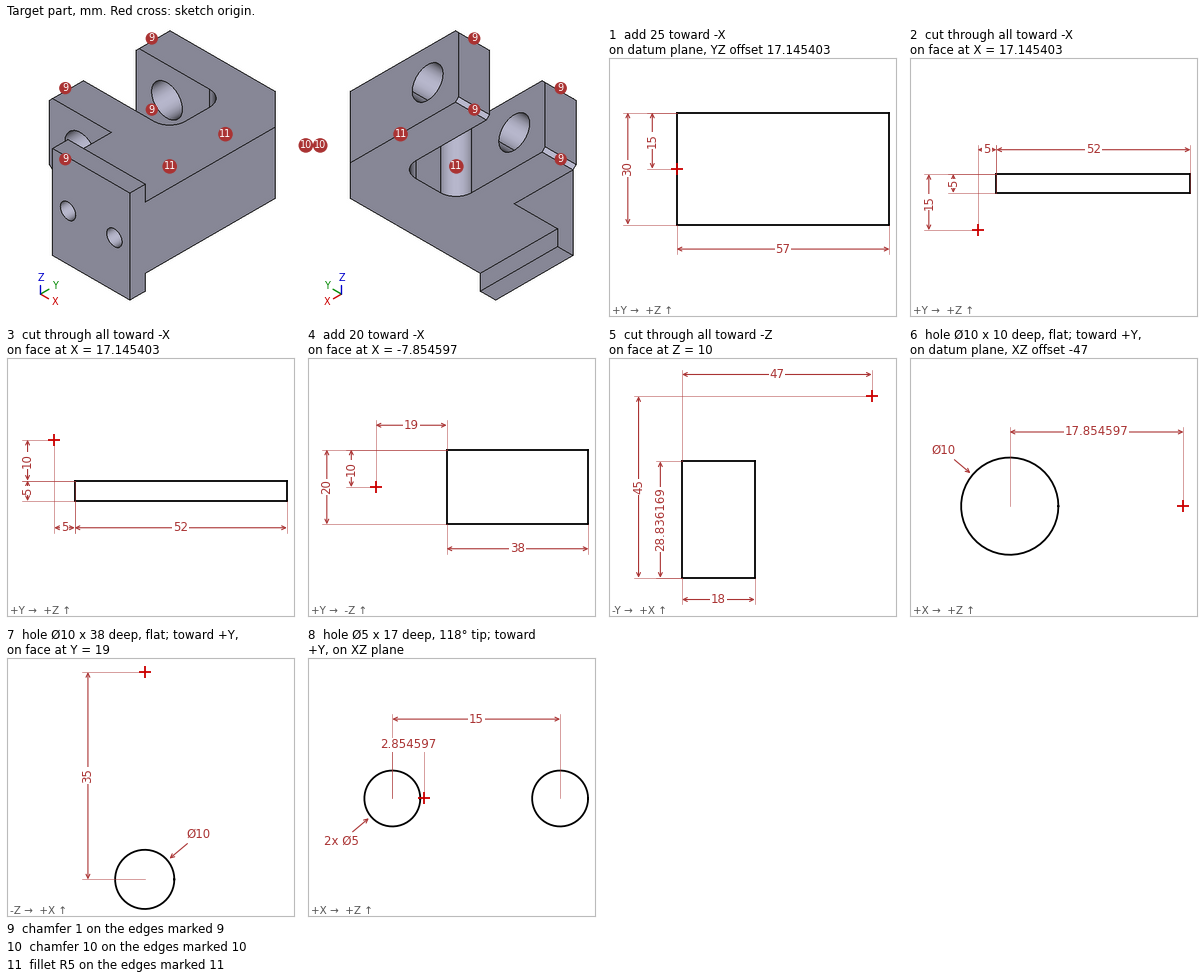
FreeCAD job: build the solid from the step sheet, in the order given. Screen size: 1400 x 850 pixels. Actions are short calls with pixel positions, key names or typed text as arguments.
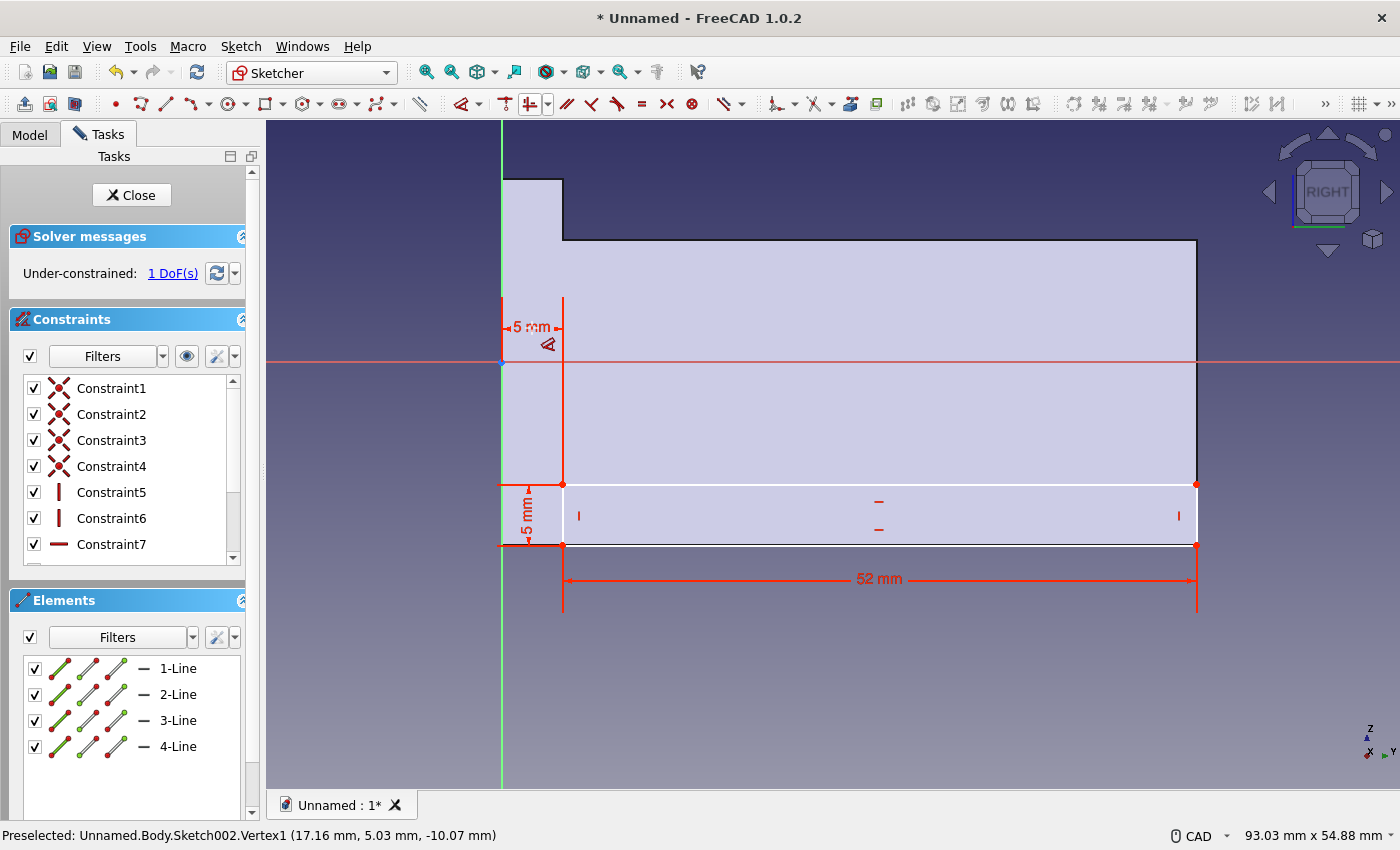
click(563, 485)
click(468, 424)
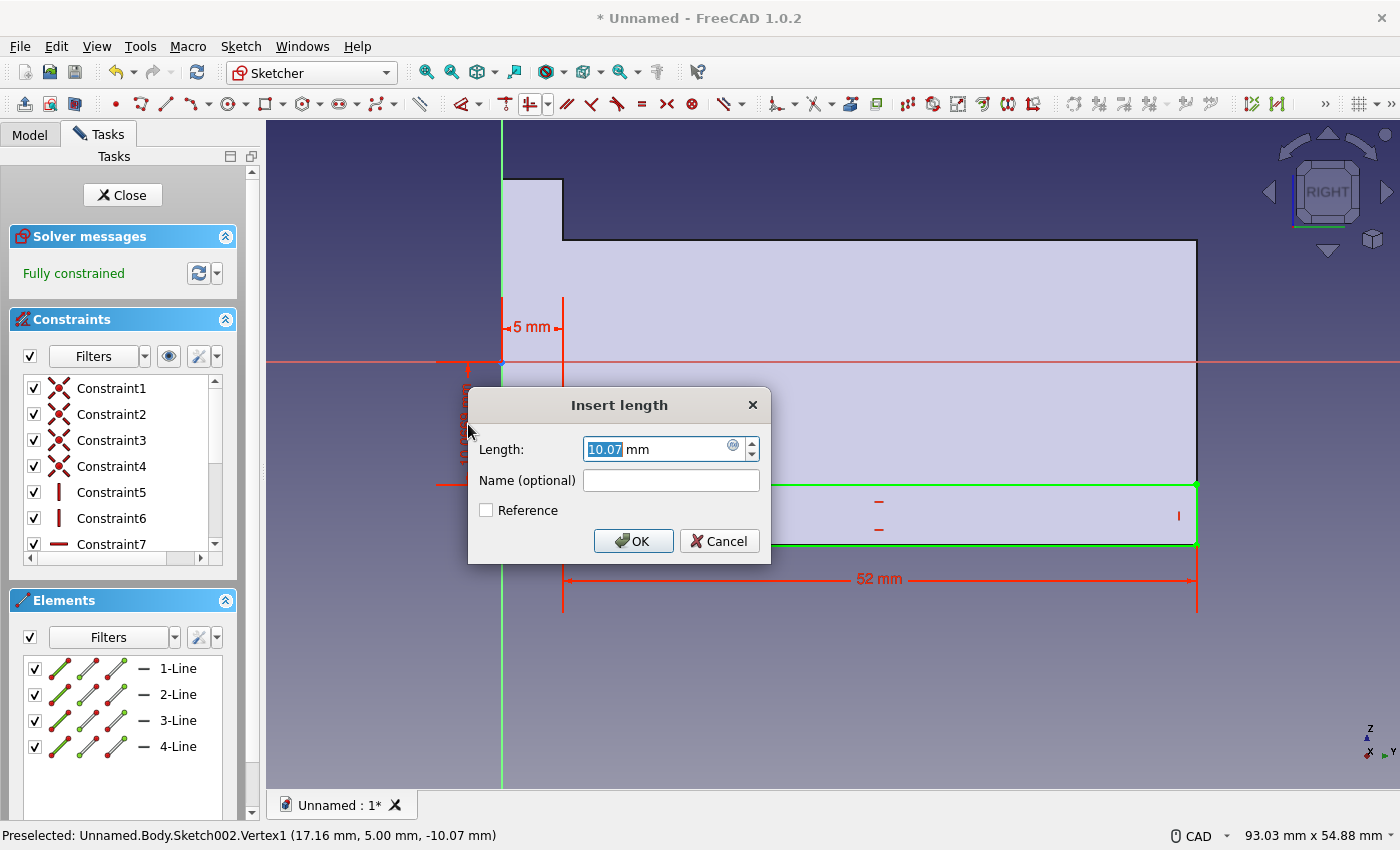
text(10)
key(Return)
key(Escape)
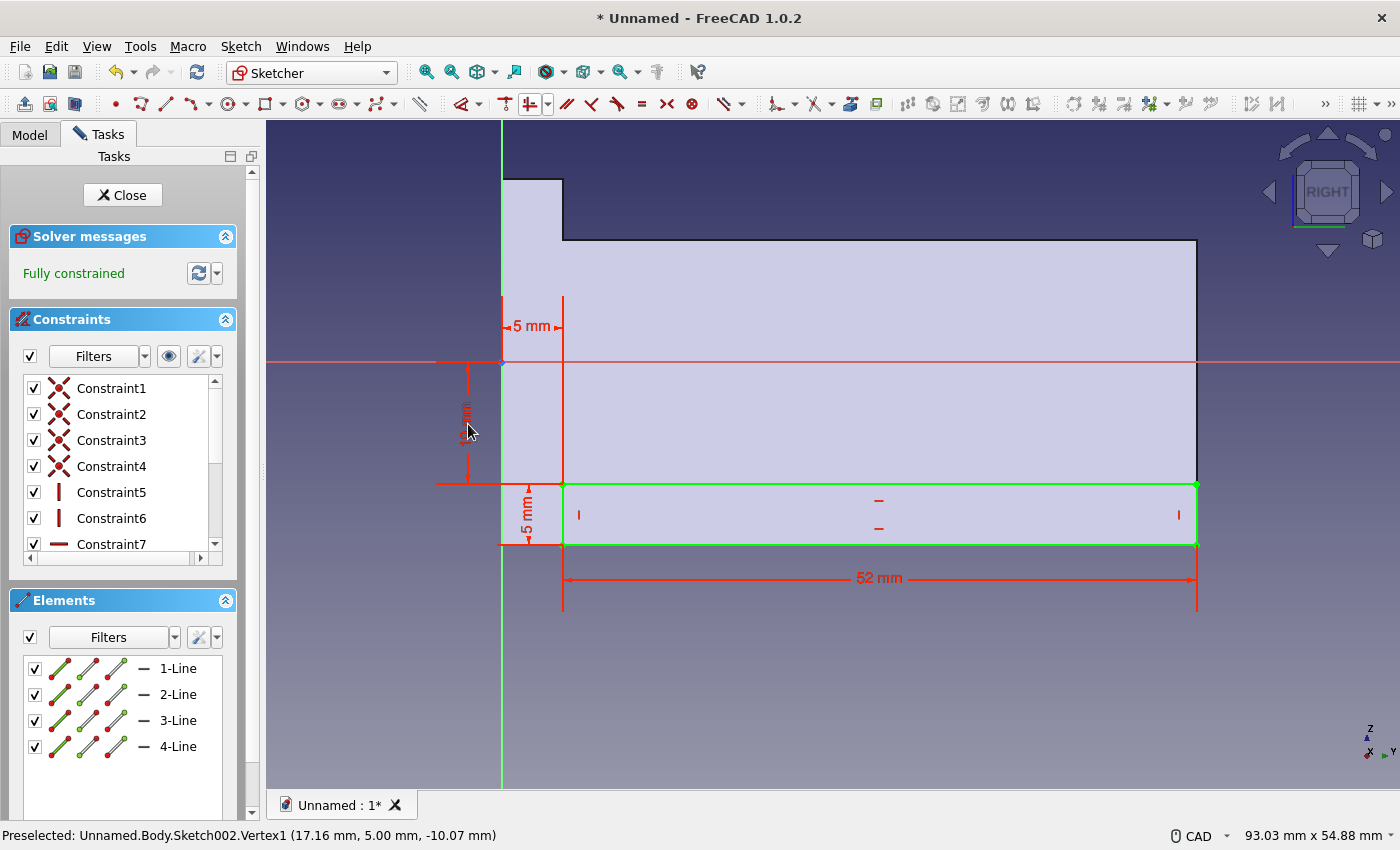
click(123, 195)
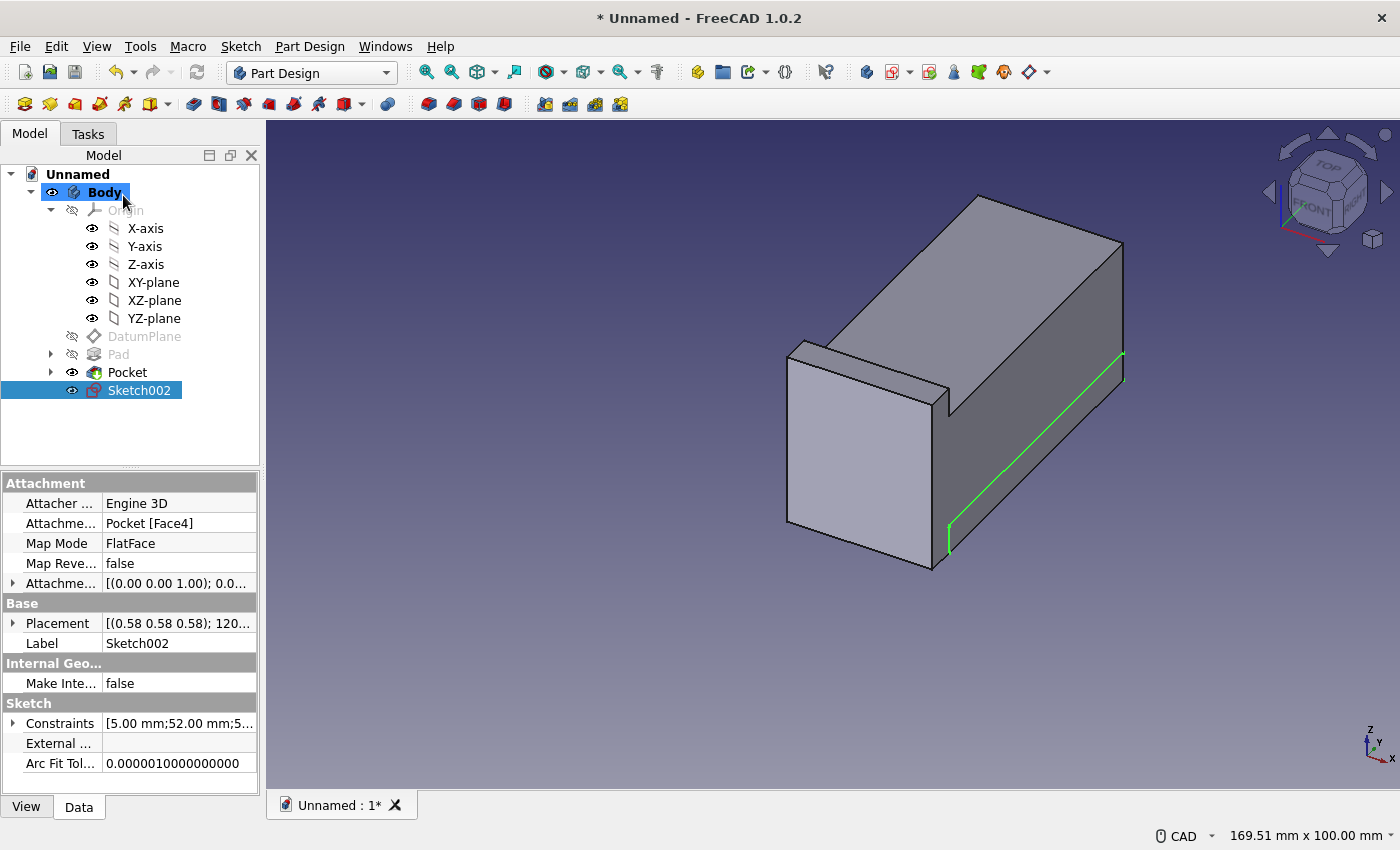
click(194, 104)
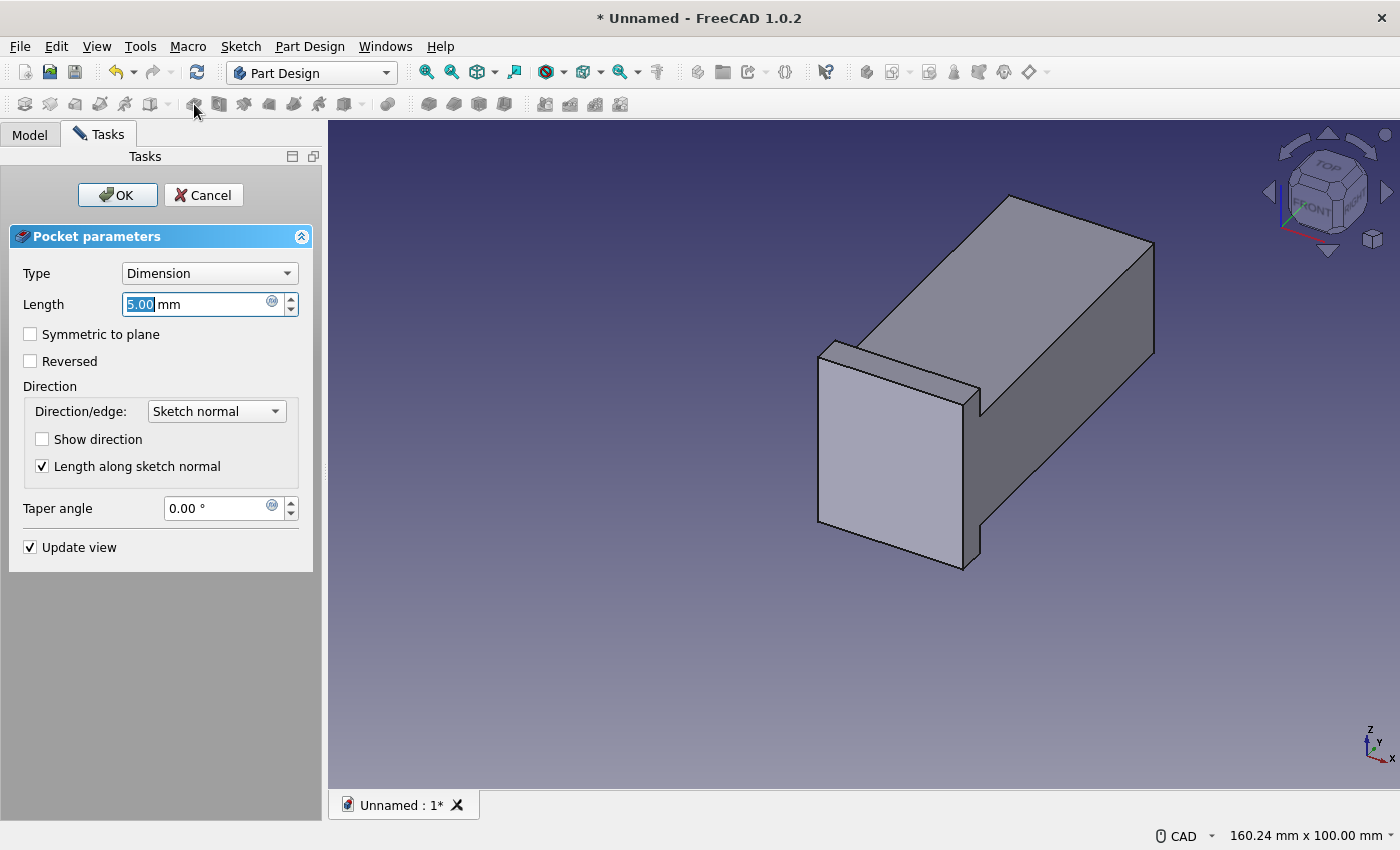
click(210, 274)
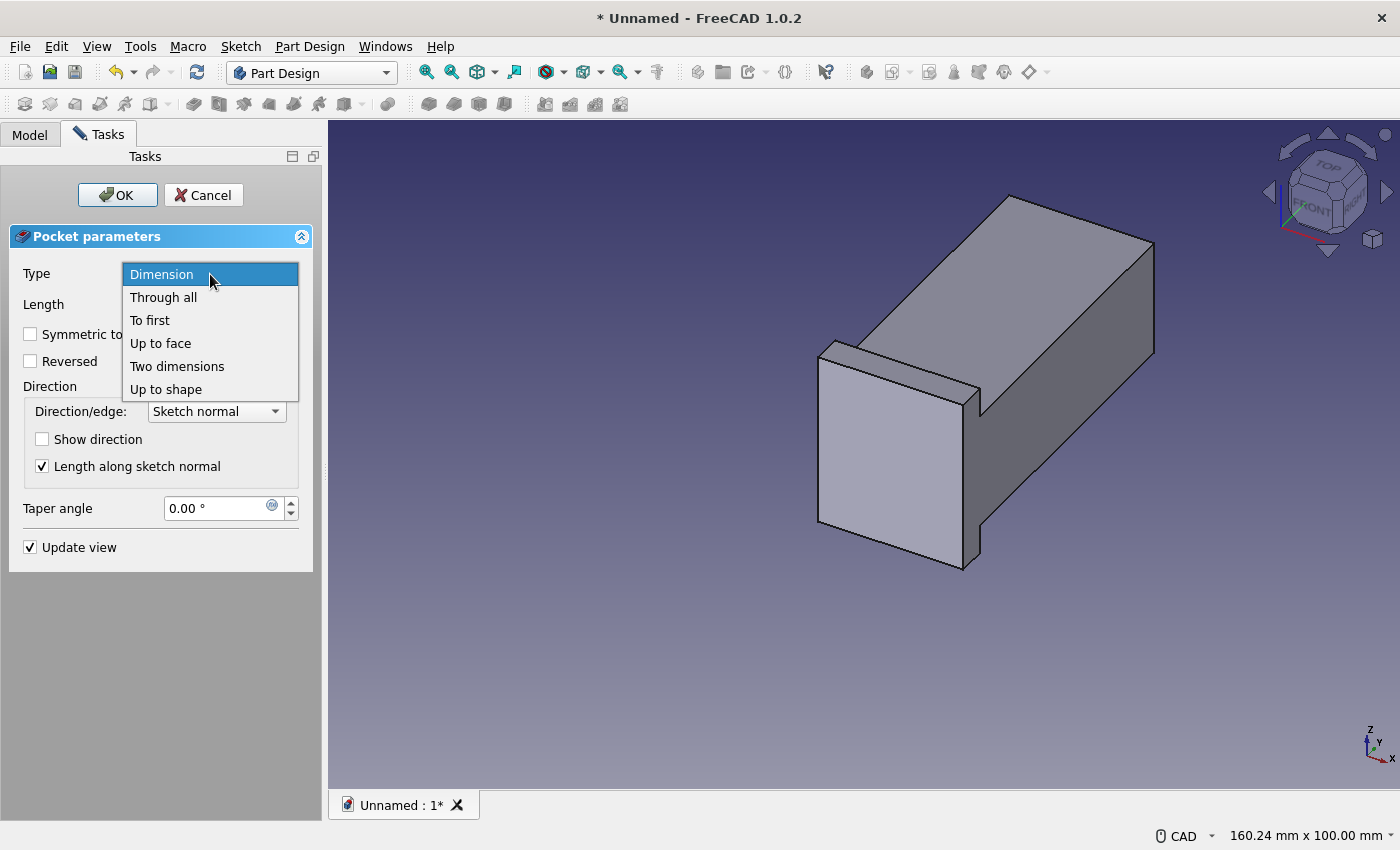
click(208, 298)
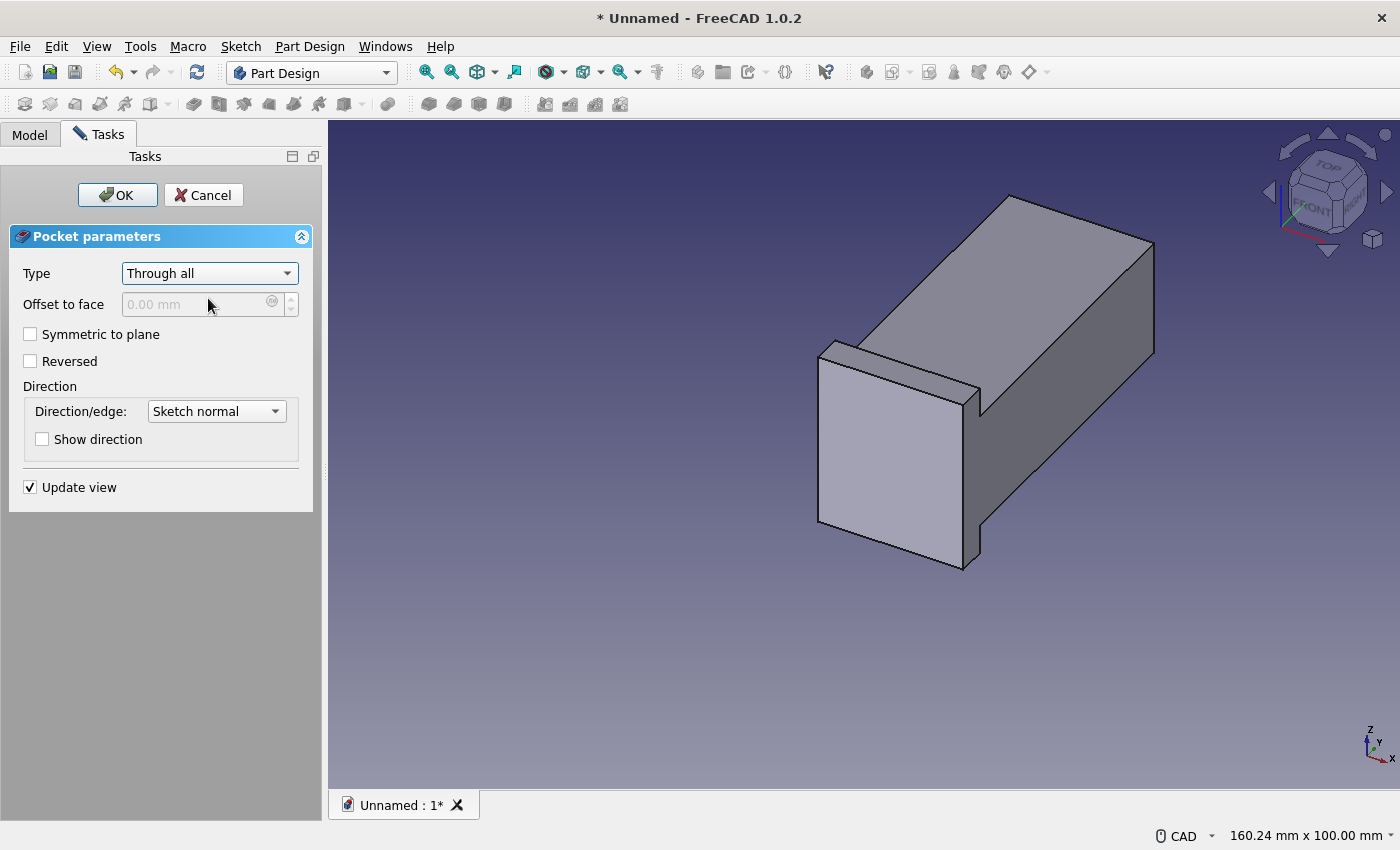
click(118, 195)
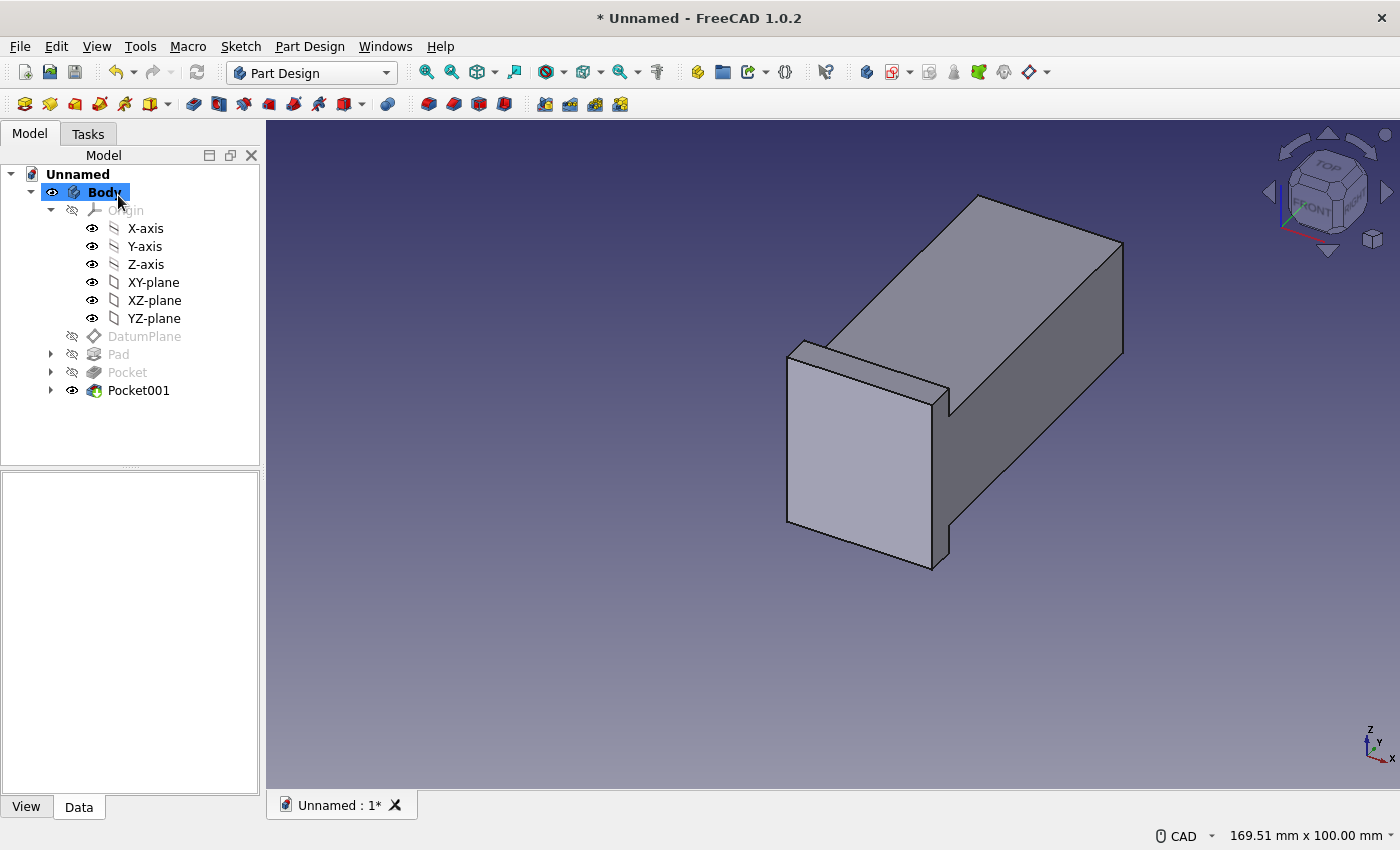
key(6)